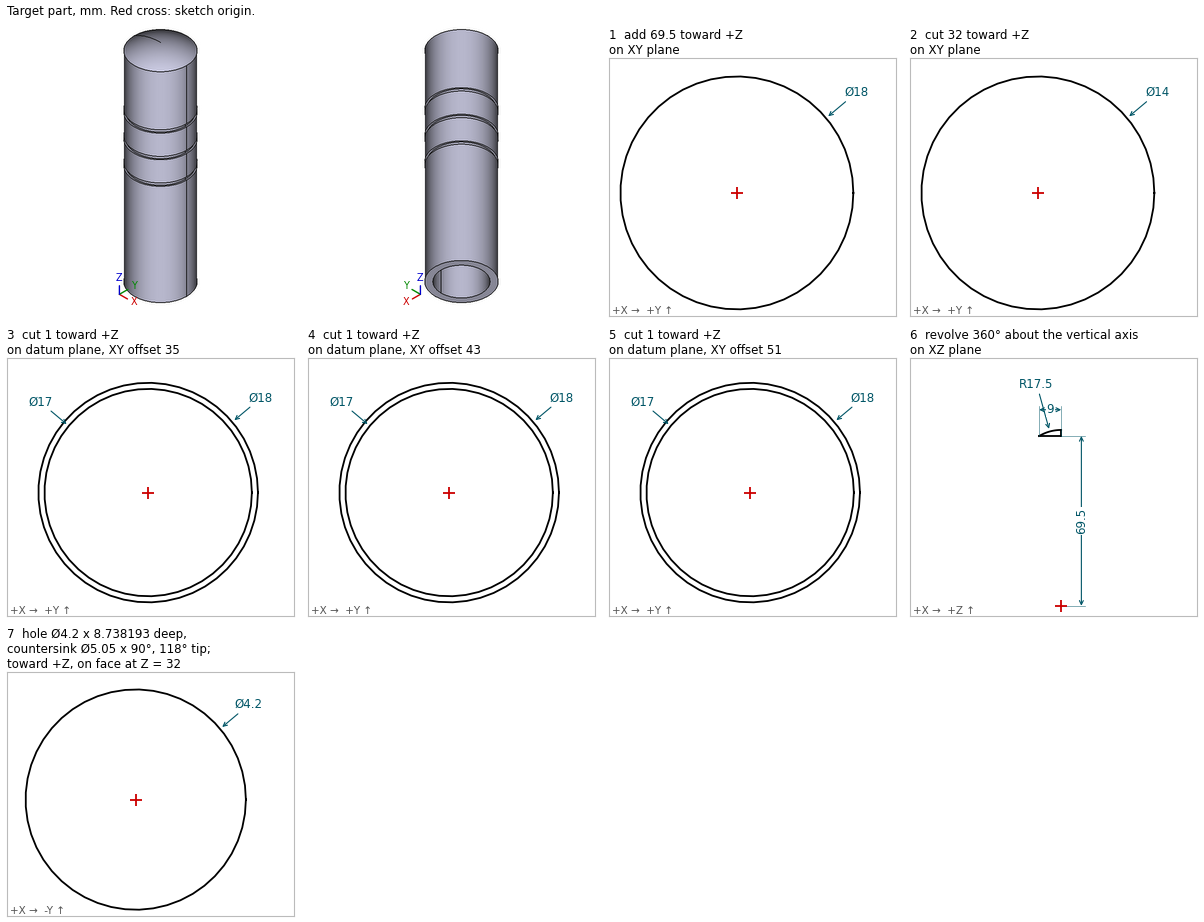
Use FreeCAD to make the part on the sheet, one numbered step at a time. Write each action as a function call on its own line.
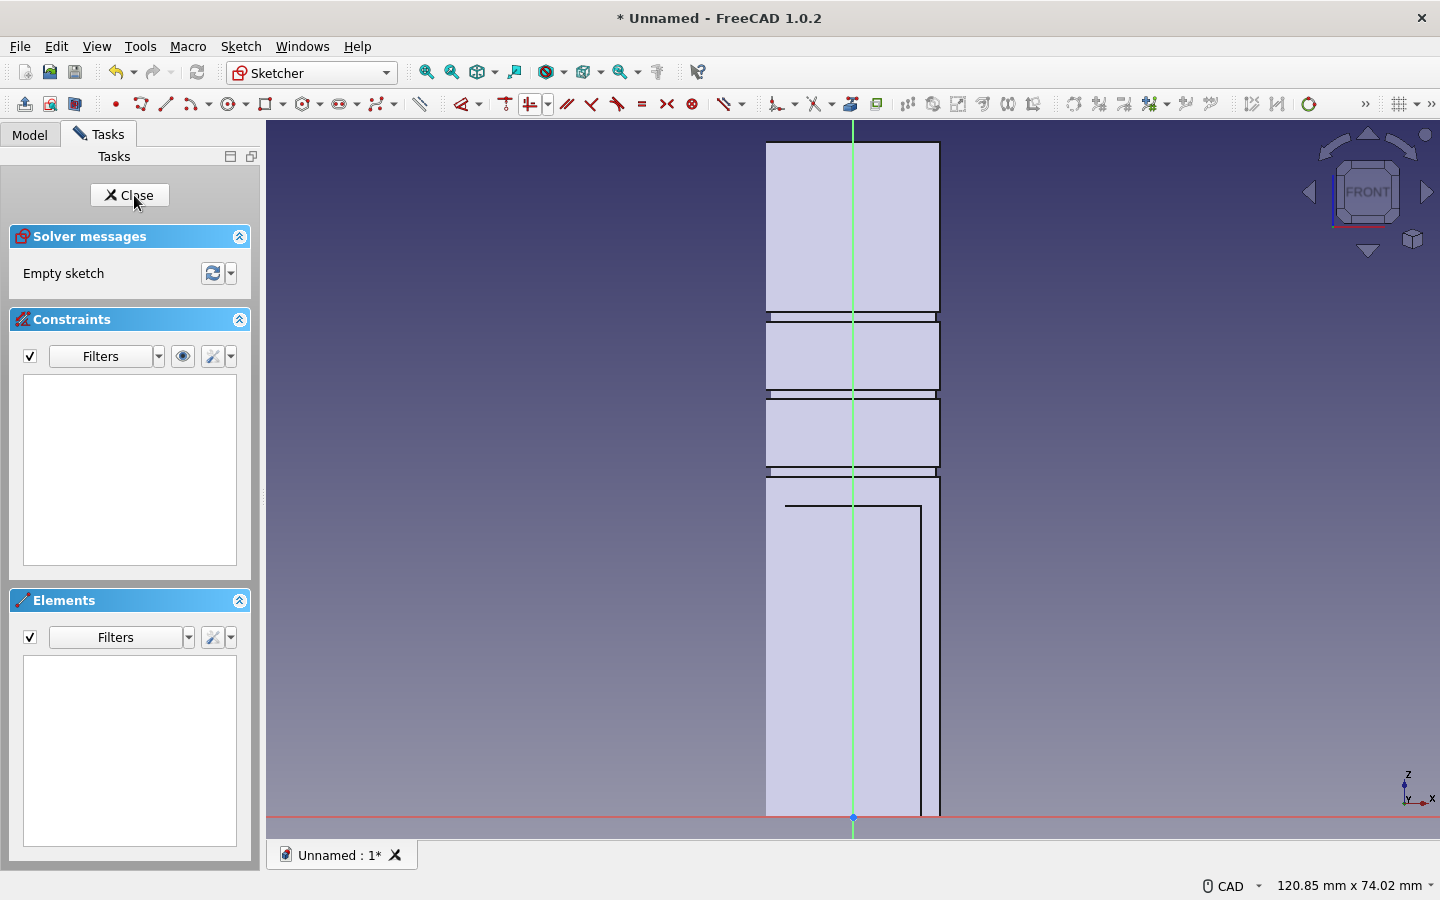
scroll(784, 480, down, 5)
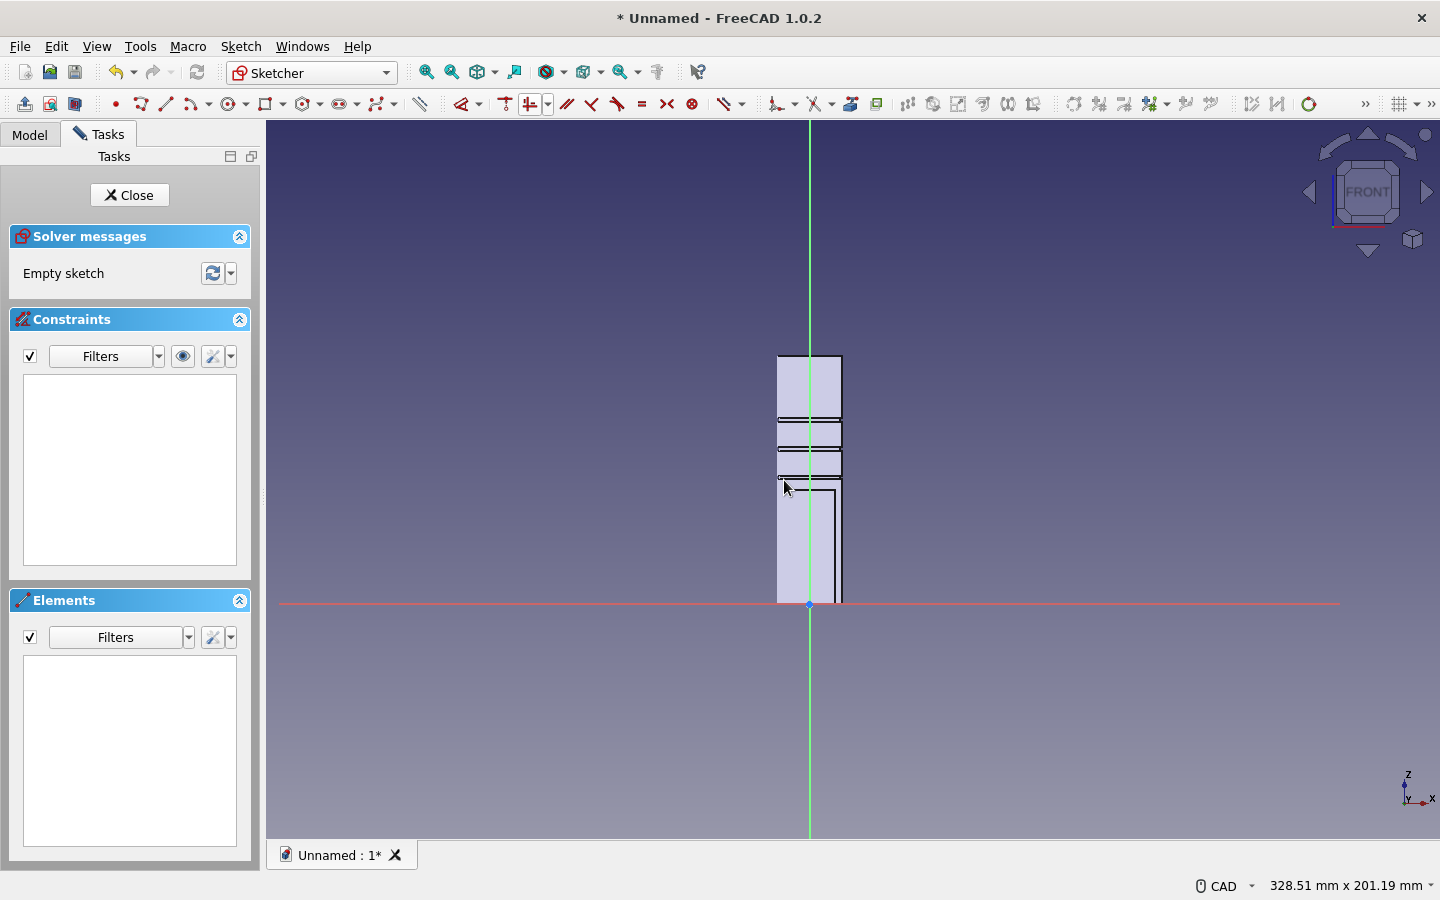
scroll(794, 345, up, 15)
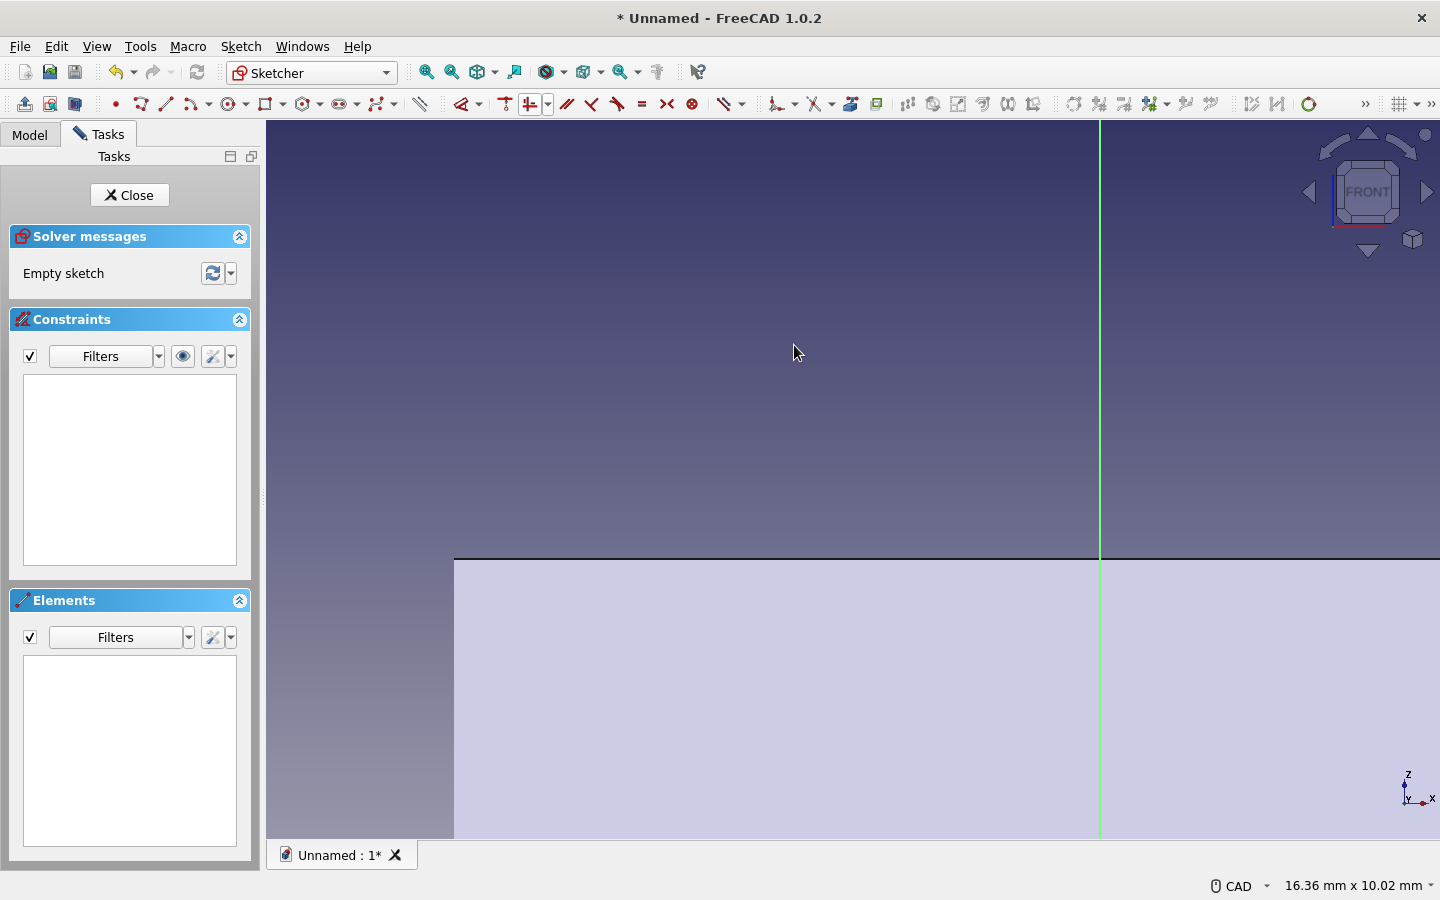
key(g)
key(m)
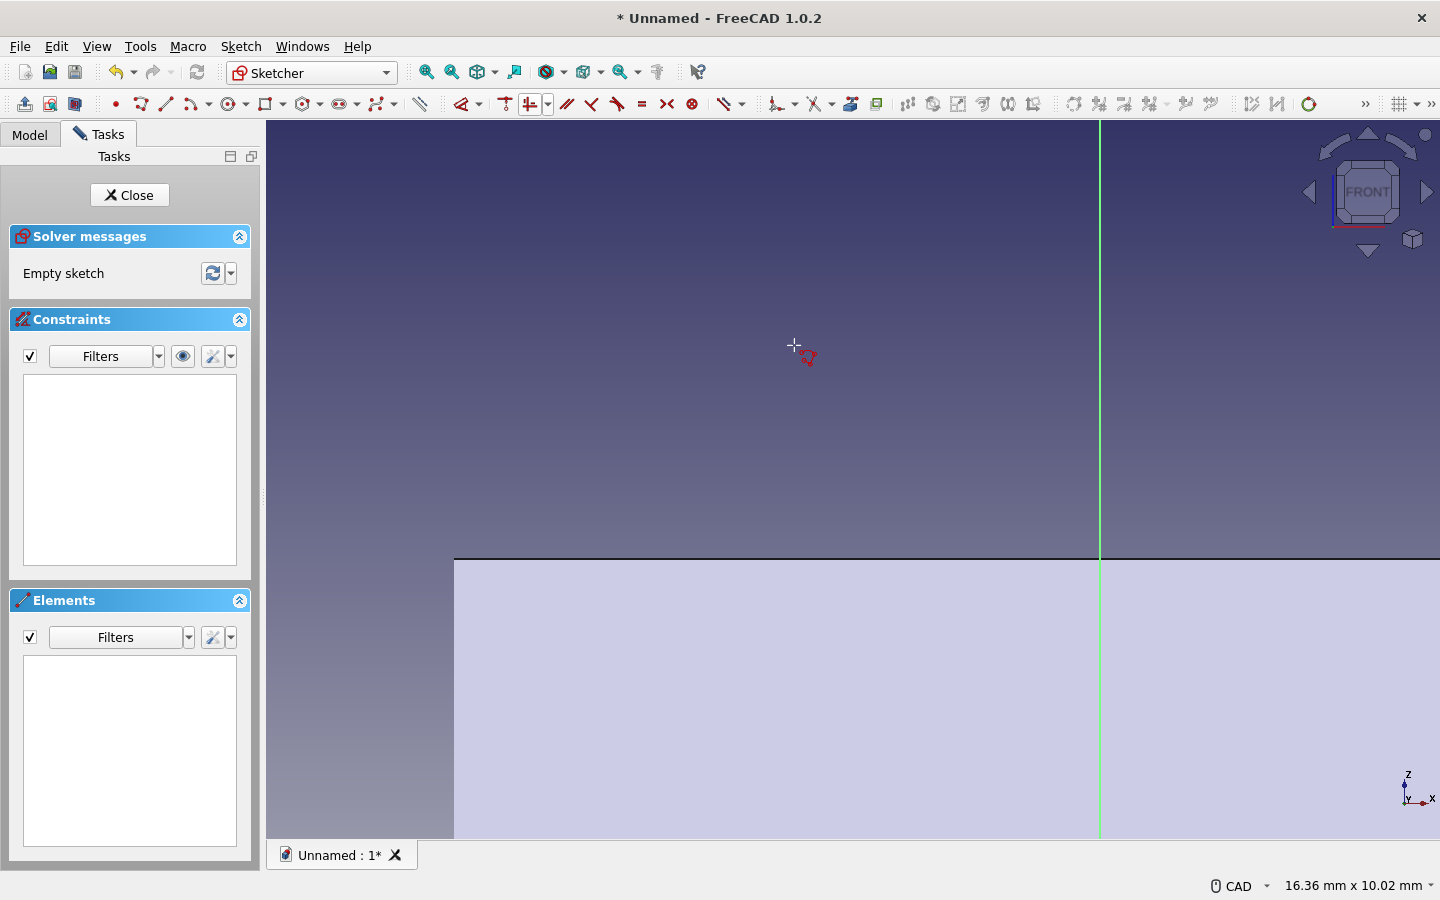
click(1100, 380)
click(1091, 559)
click(454, 559)
right_click(454, 559)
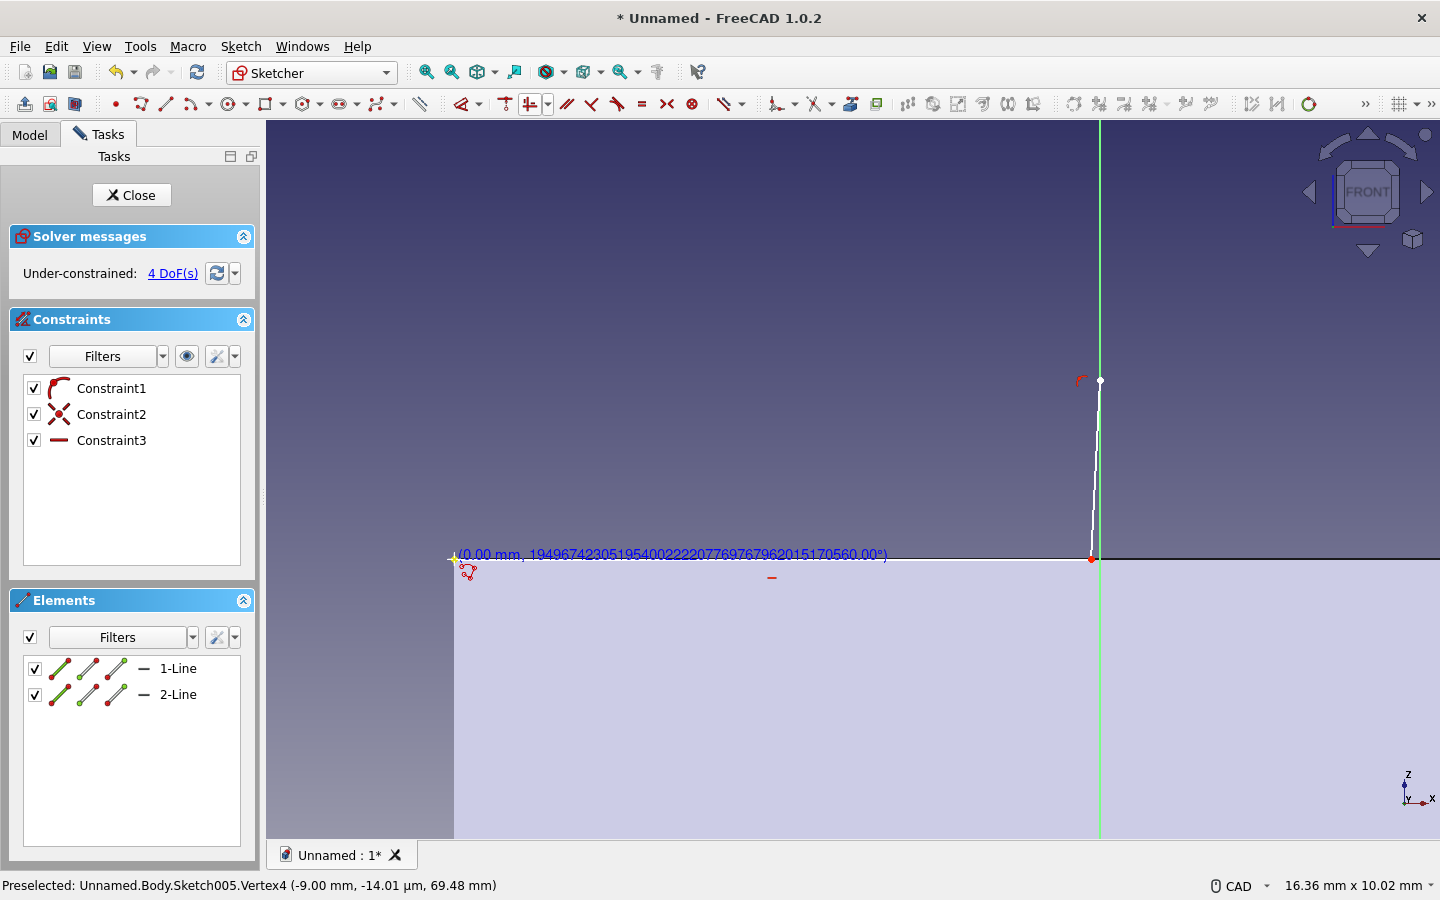
key(g)
key(3)
key(a)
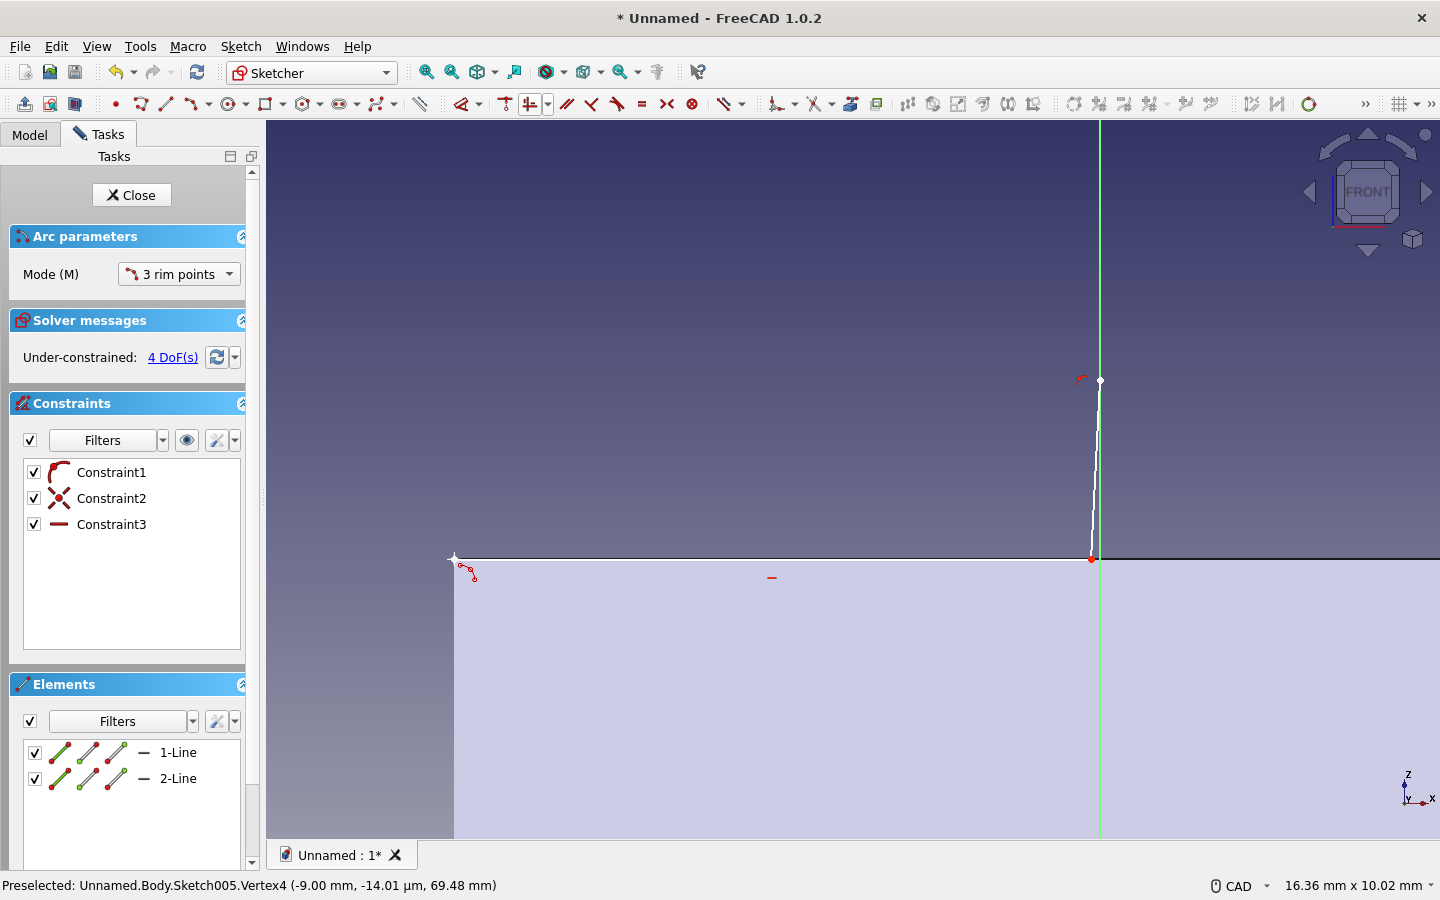
click(454, 560)
click(1100, 381)
click(765, 426)
key(Escape)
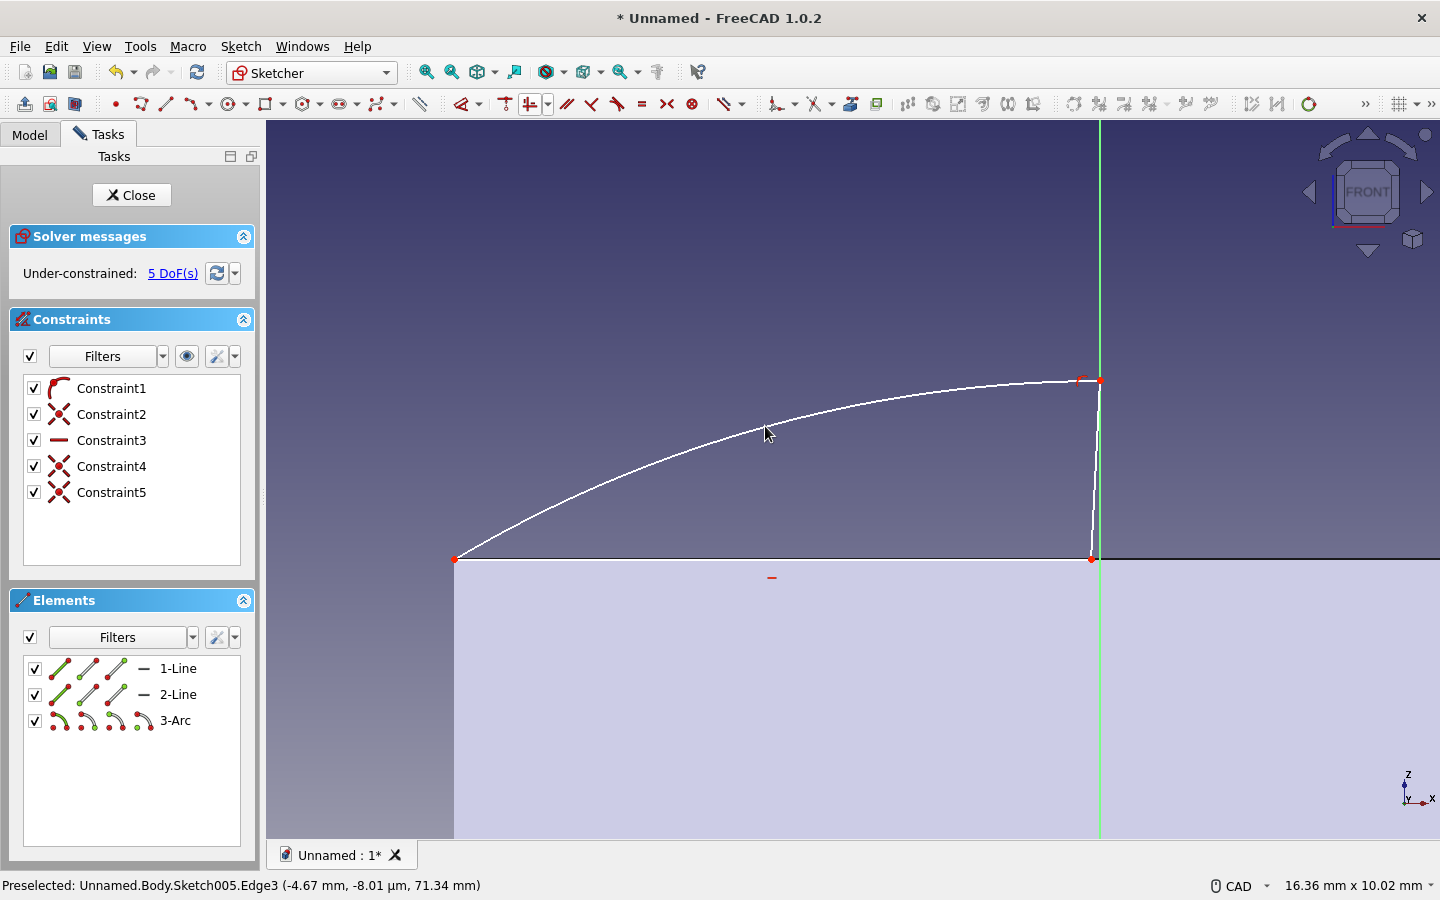
click(1097, 435)